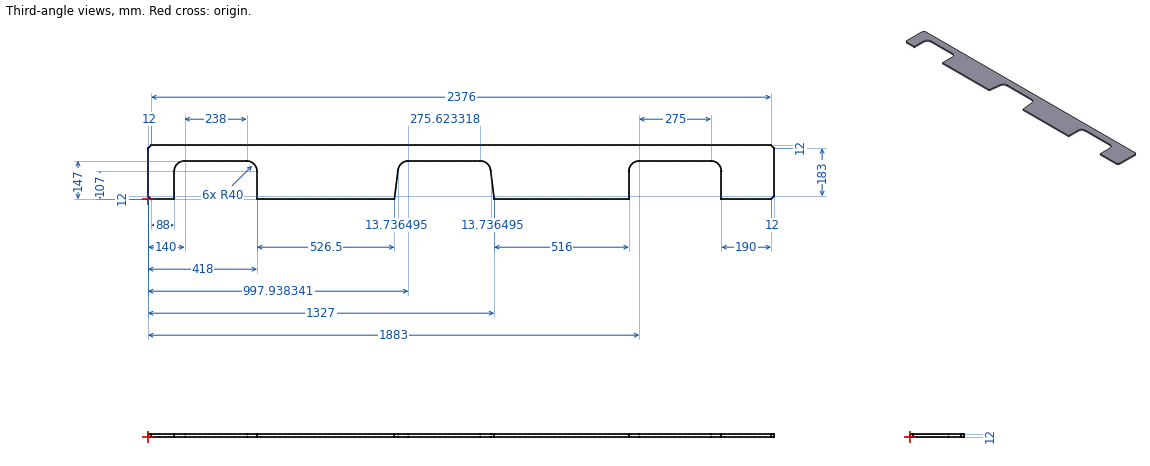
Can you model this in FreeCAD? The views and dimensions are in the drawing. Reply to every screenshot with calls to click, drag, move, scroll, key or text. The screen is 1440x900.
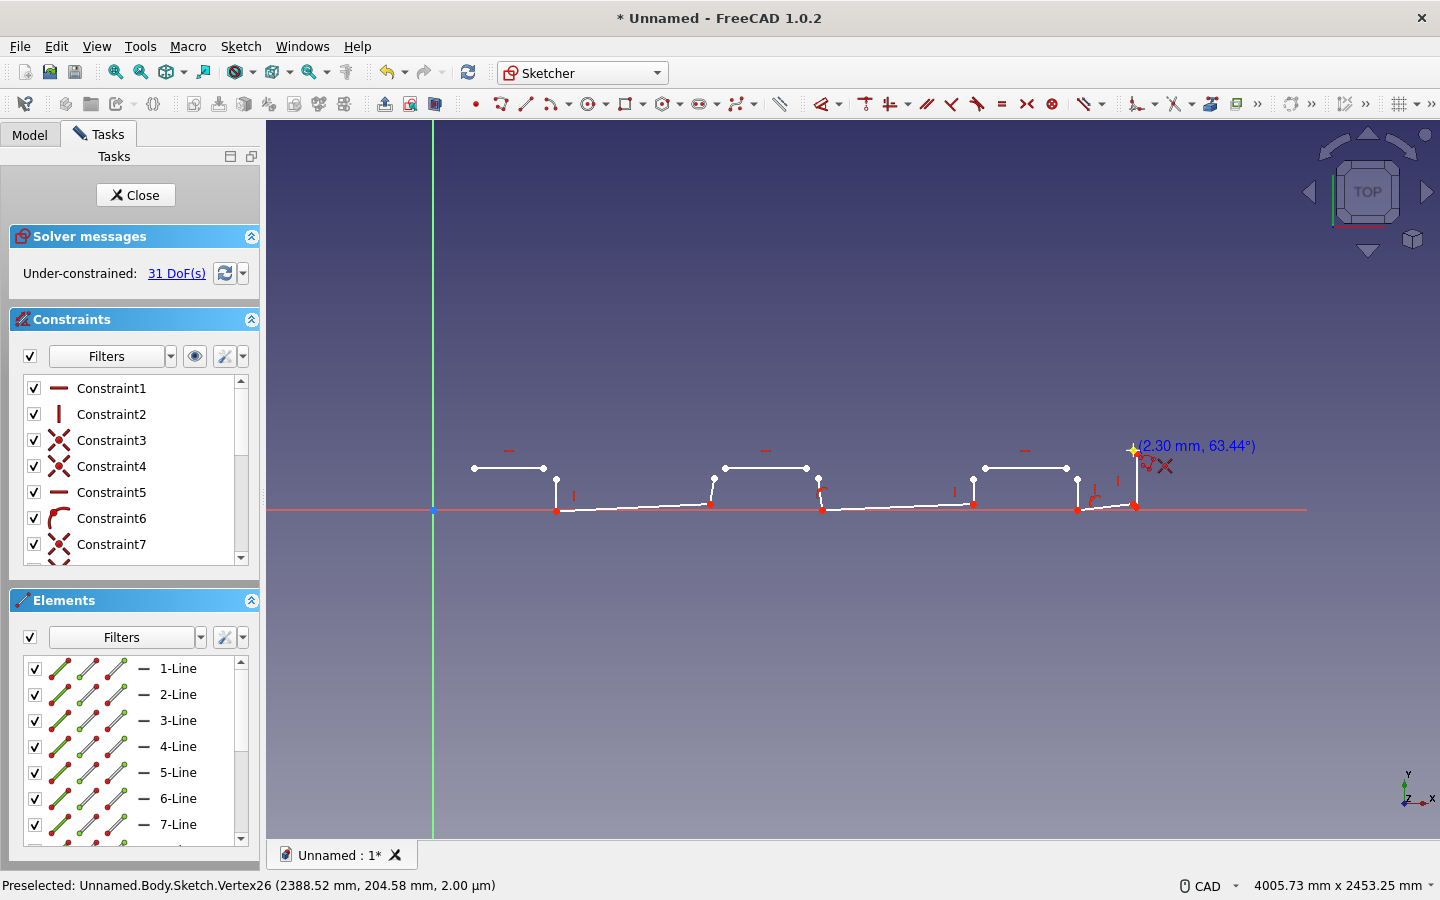
scroll(437, 450, up, 8)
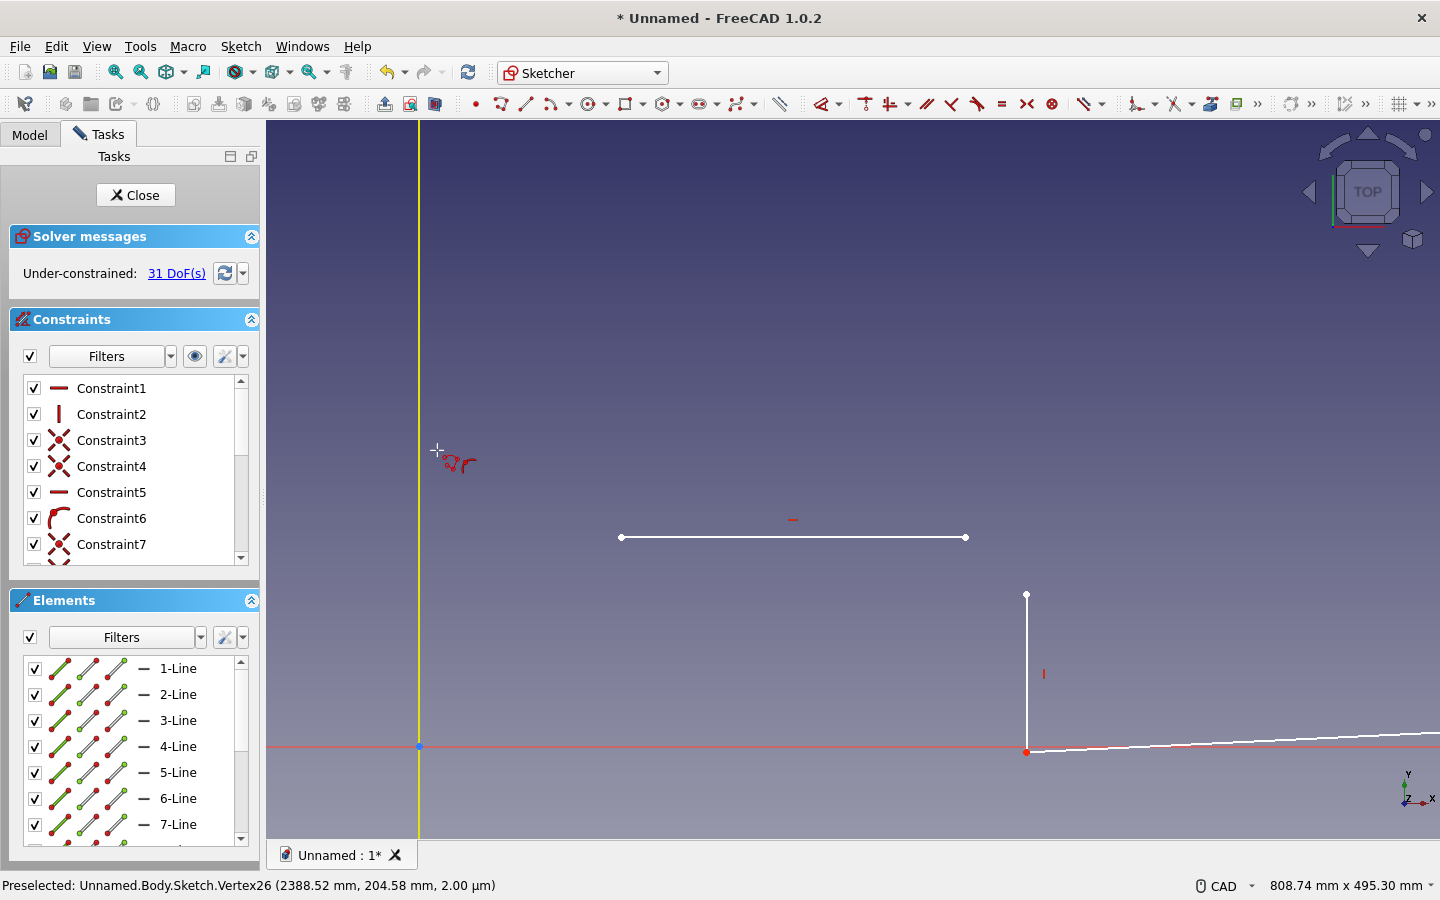
click(436, 447)
click(419, 464)
click(428, 729)
click(436, 747)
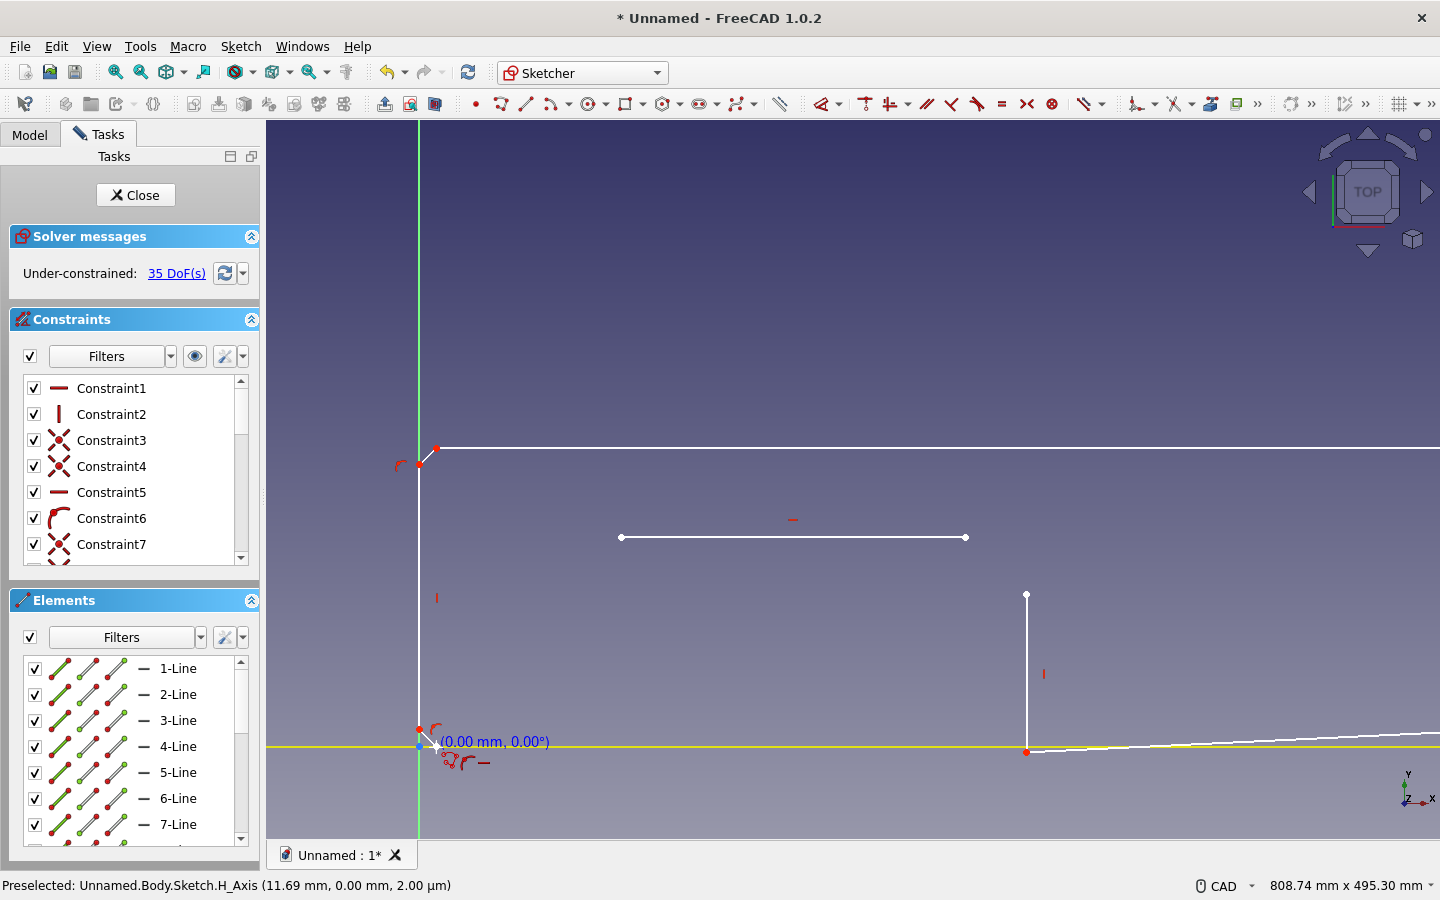
scroll(436, 450, down, 8)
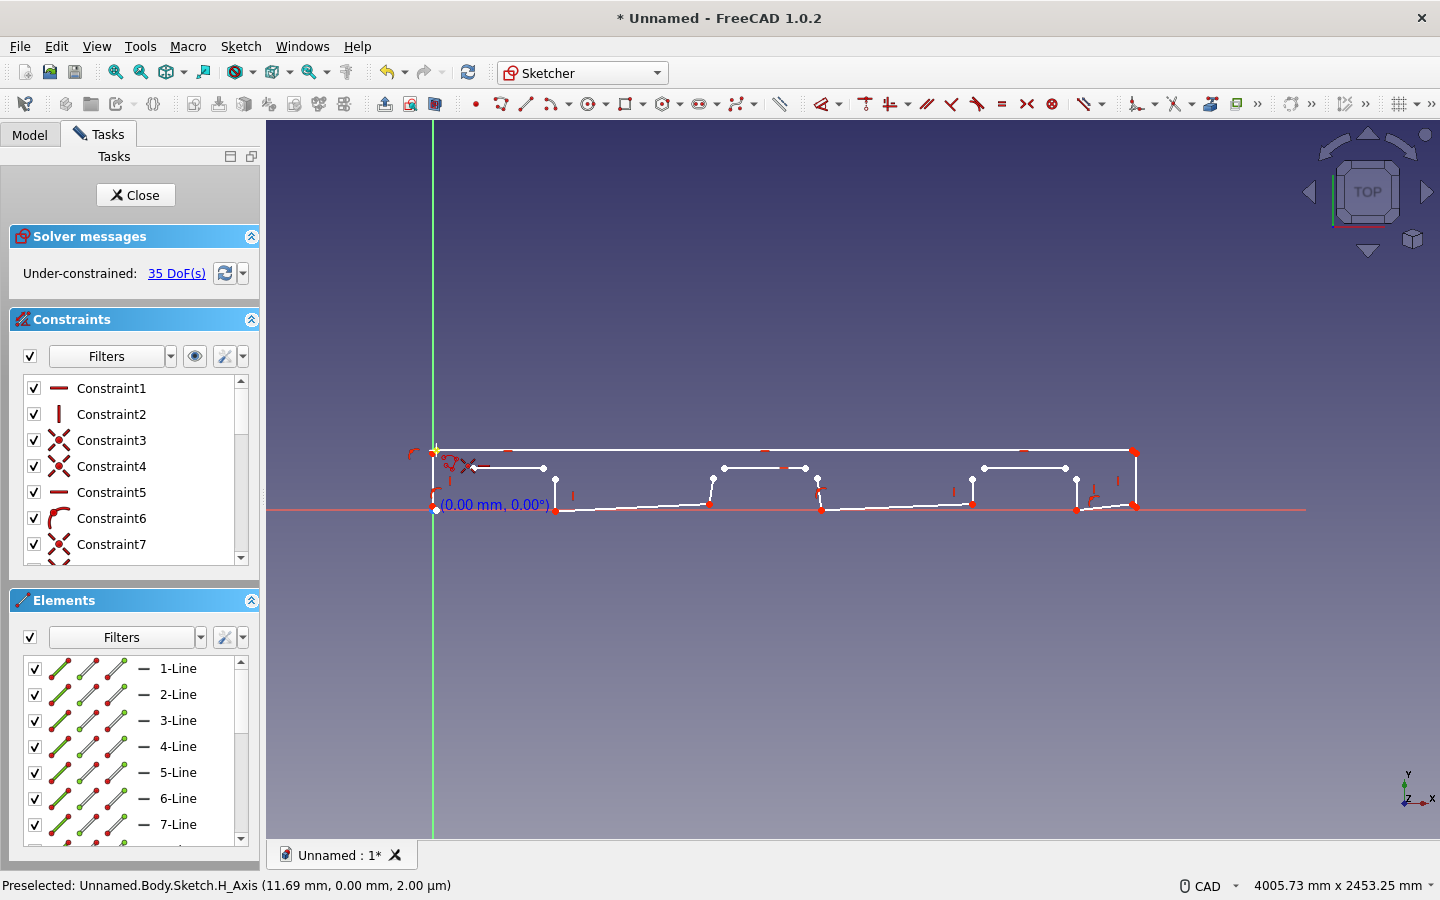
click(462, 501)
click(462, 479)
right_click(462, 479)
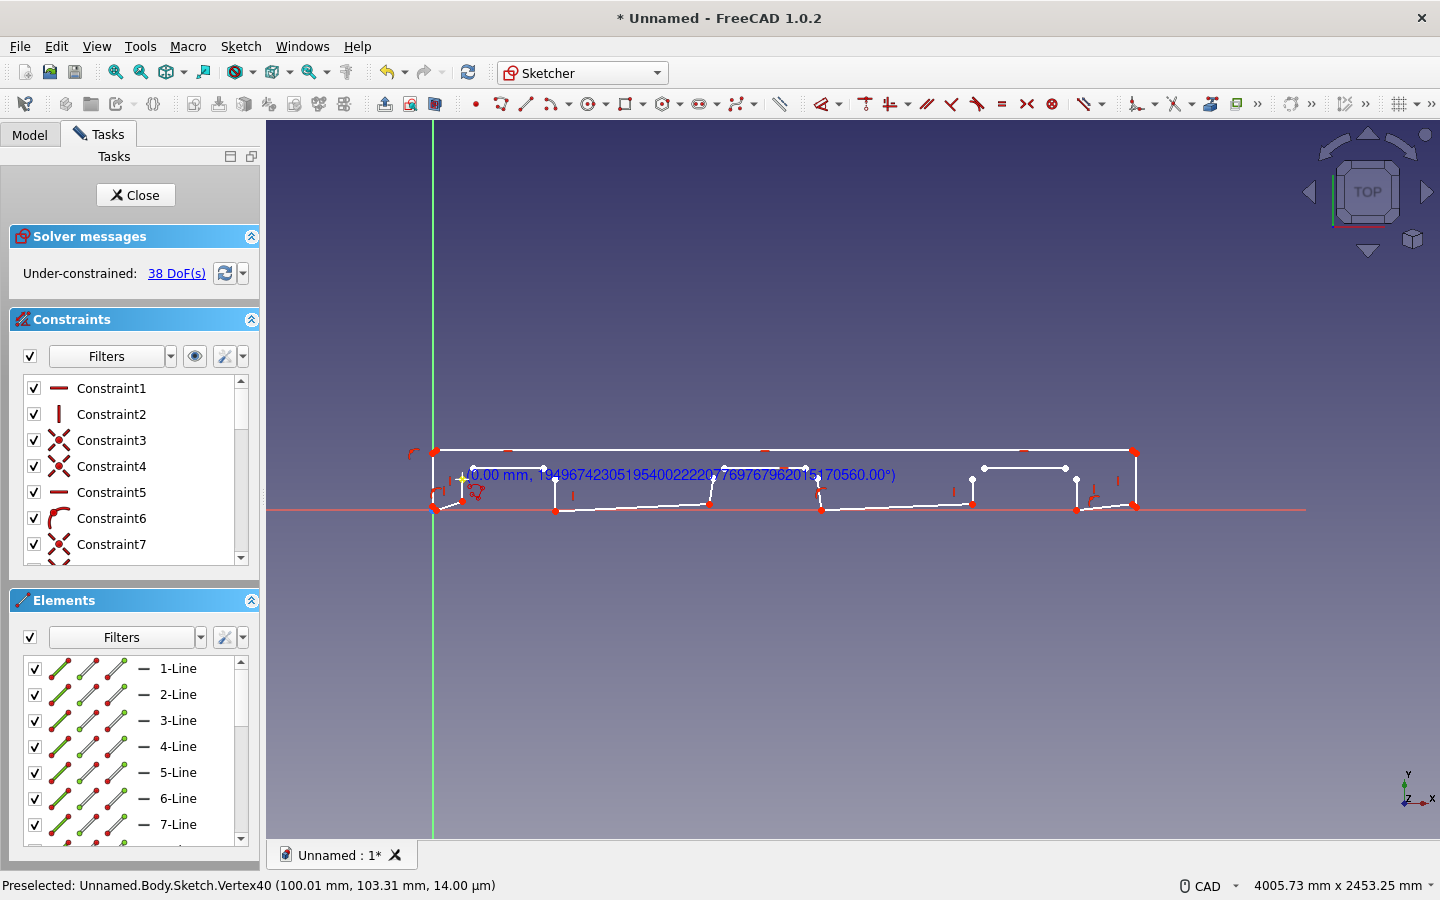
click(568, 104)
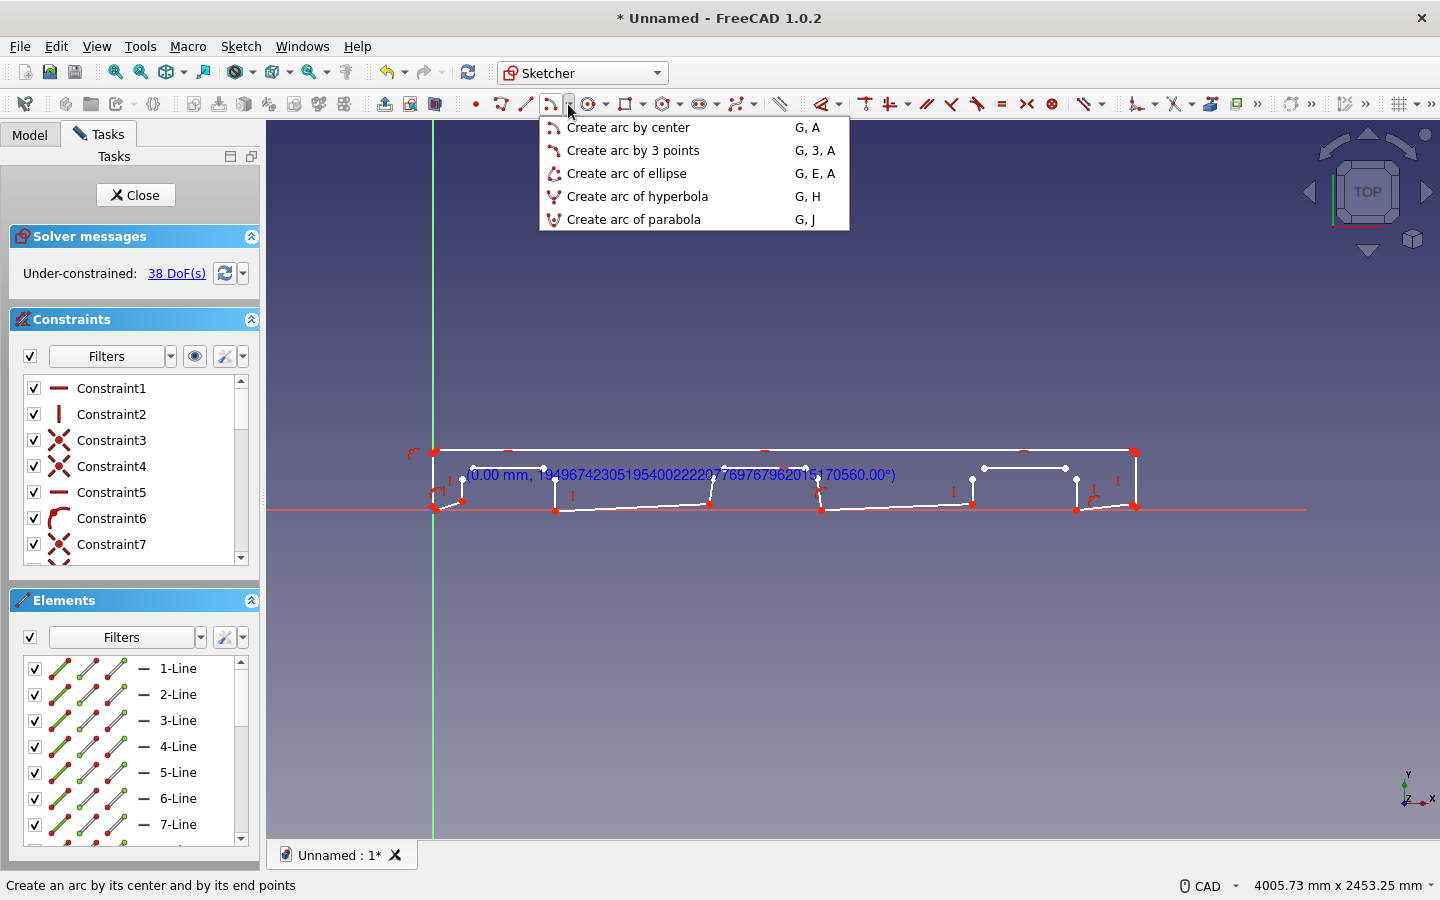
click(694, 150)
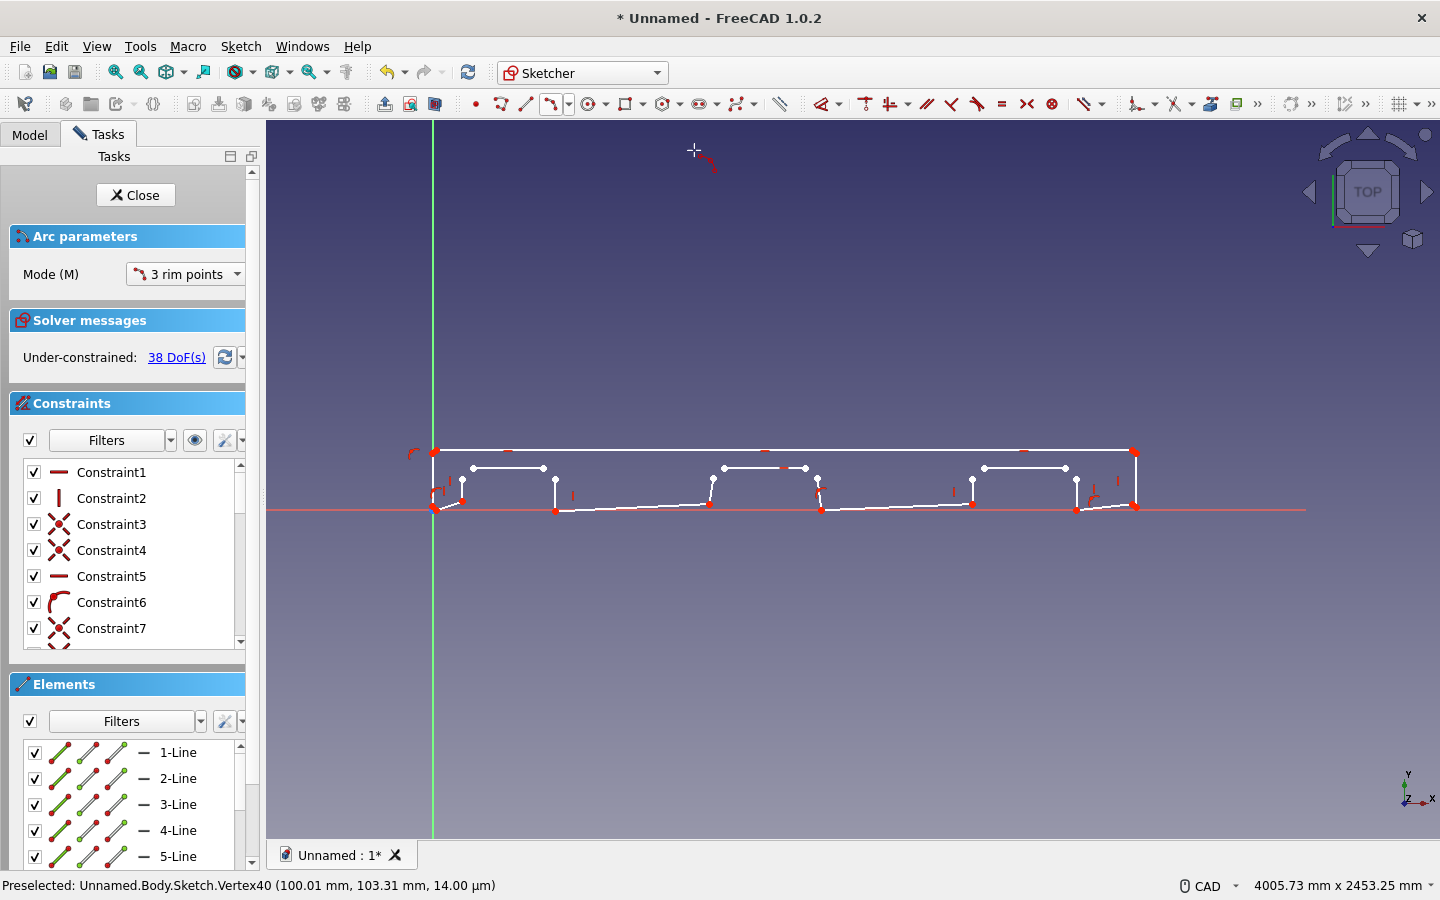
click(543, 468)
click(555, 479)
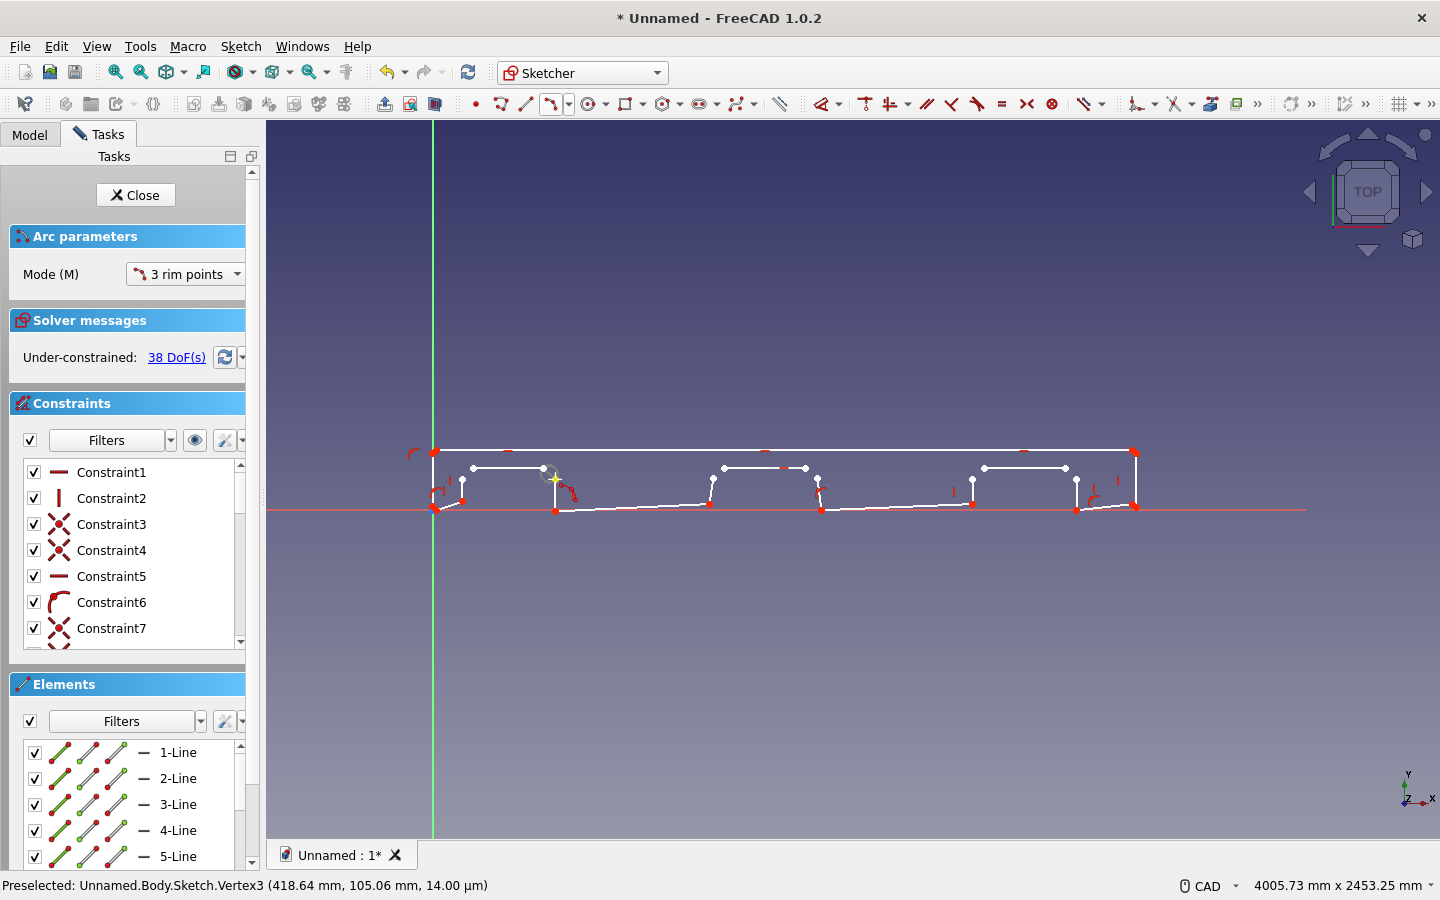
scroll(552, 471, up, 8)